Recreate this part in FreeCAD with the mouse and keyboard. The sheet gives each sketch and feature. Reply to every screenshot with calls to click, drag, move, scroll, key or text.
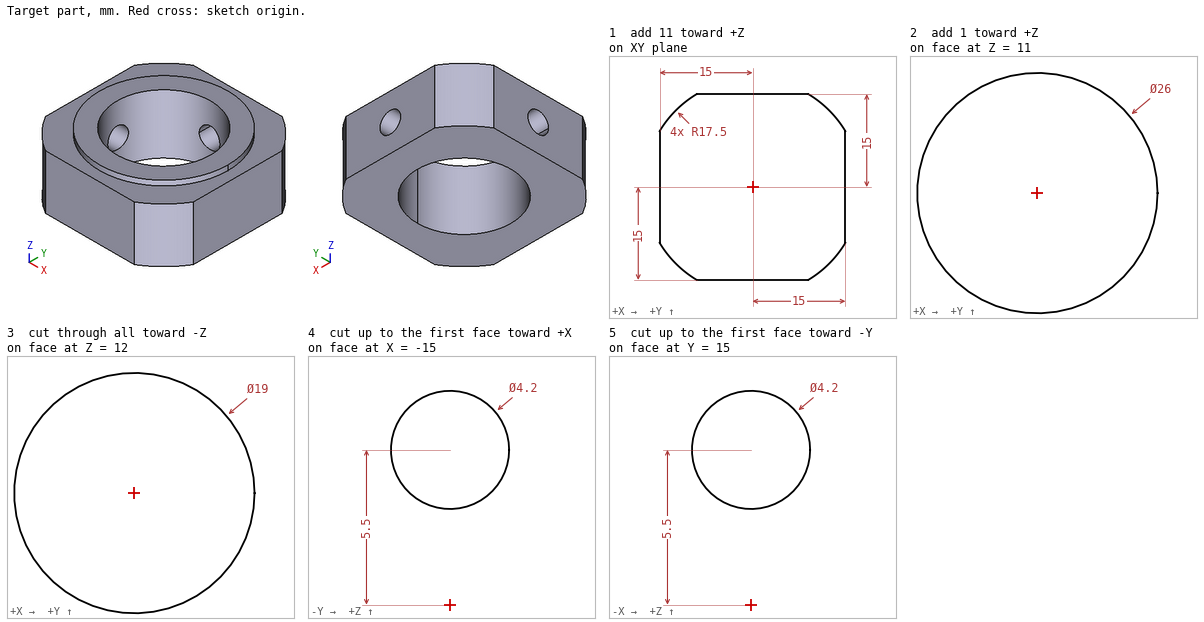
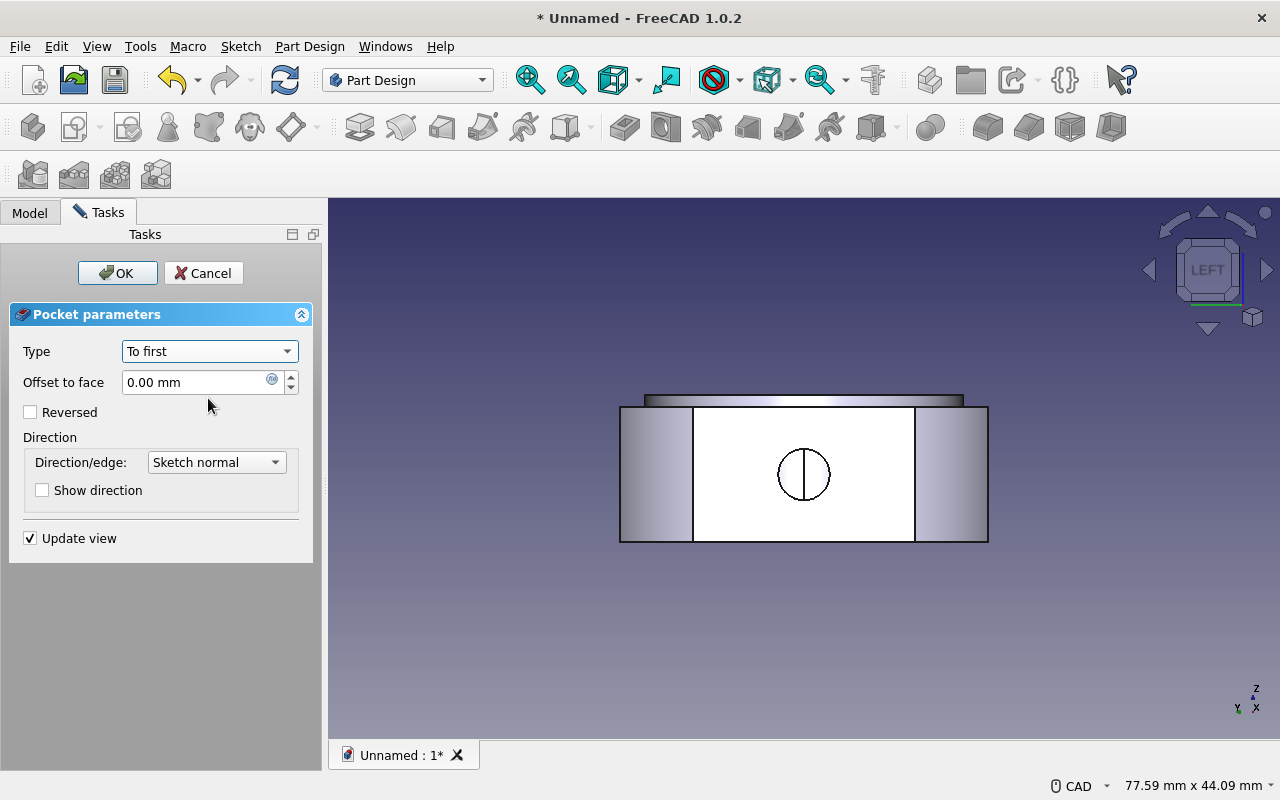
click(118, 273)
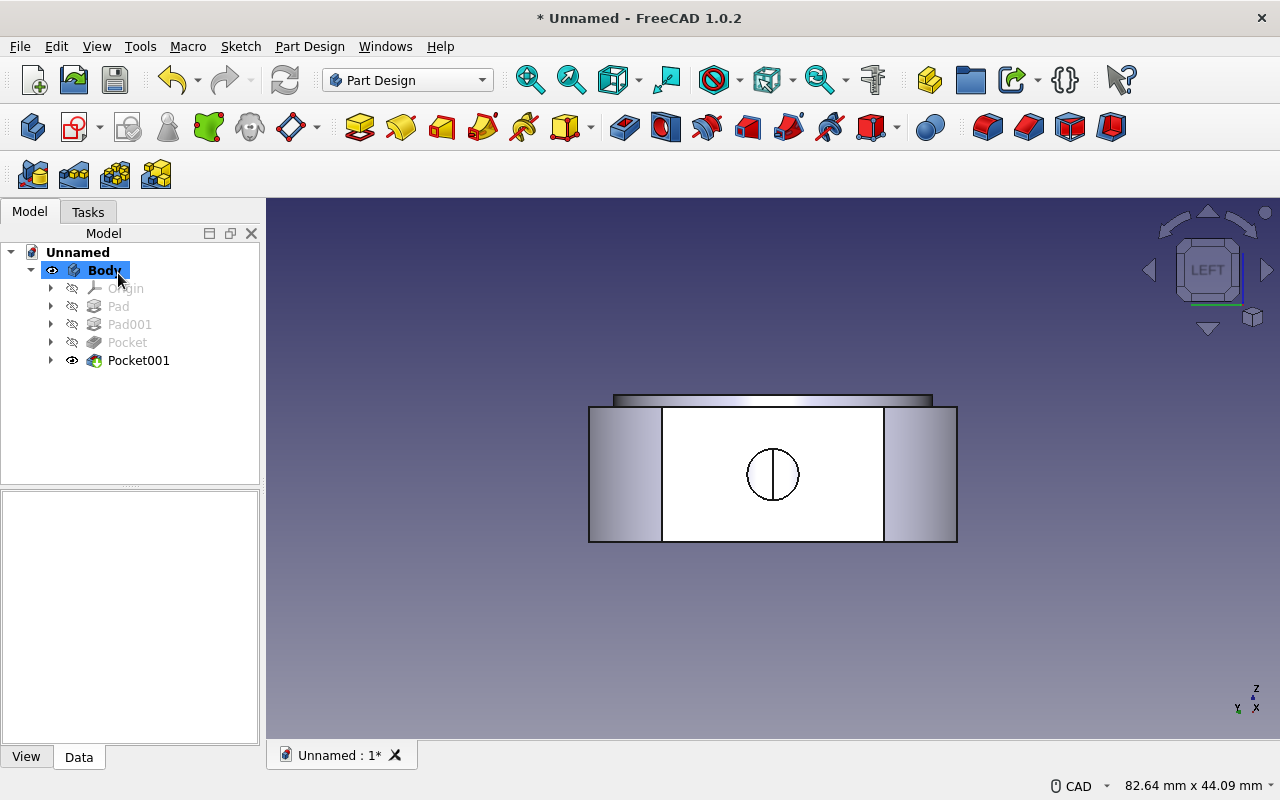
click(531, 80)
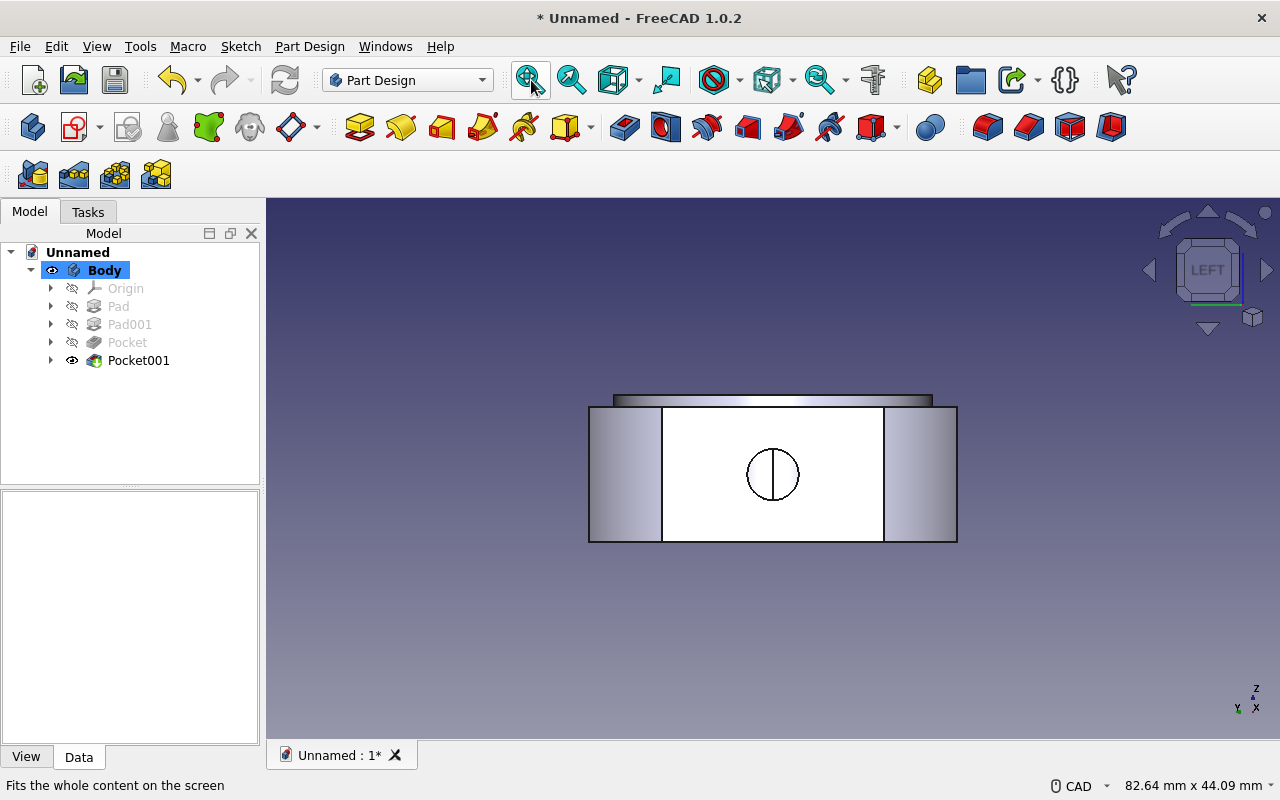
key(4)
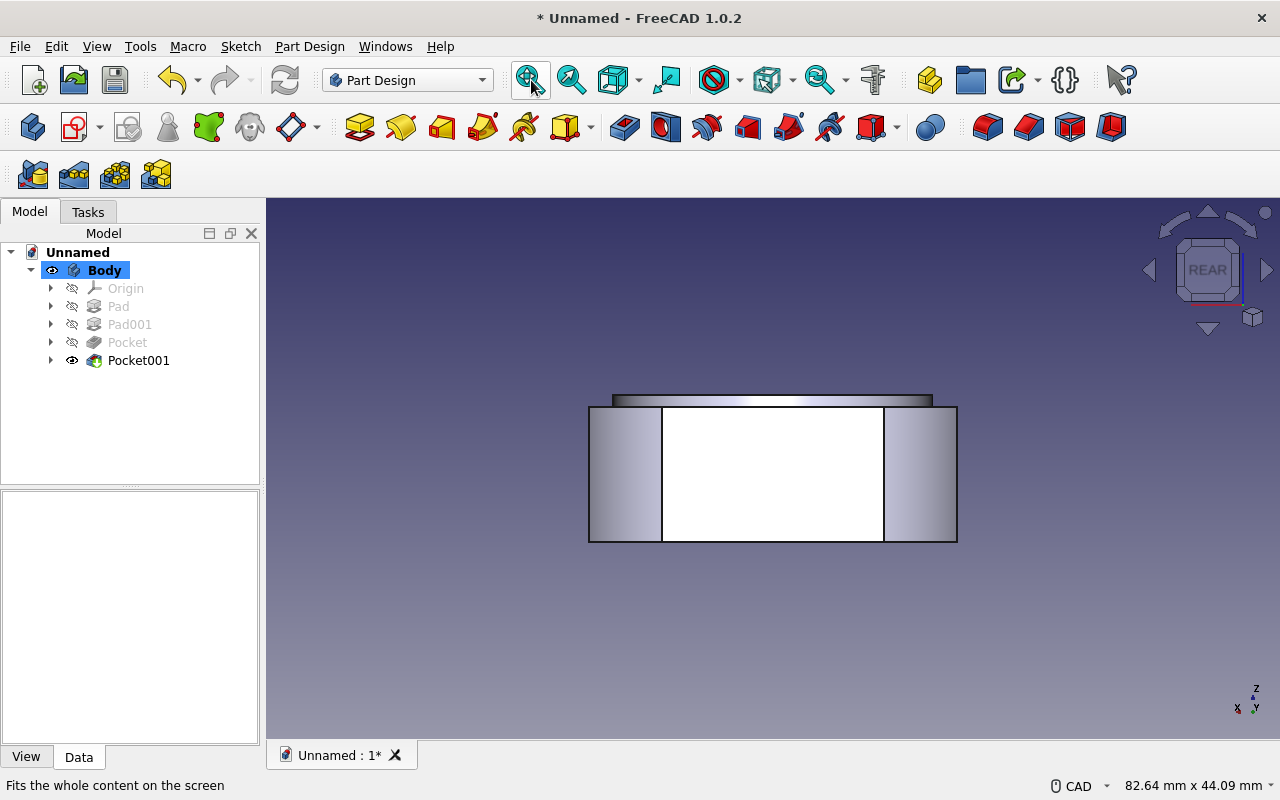
click(531, 80)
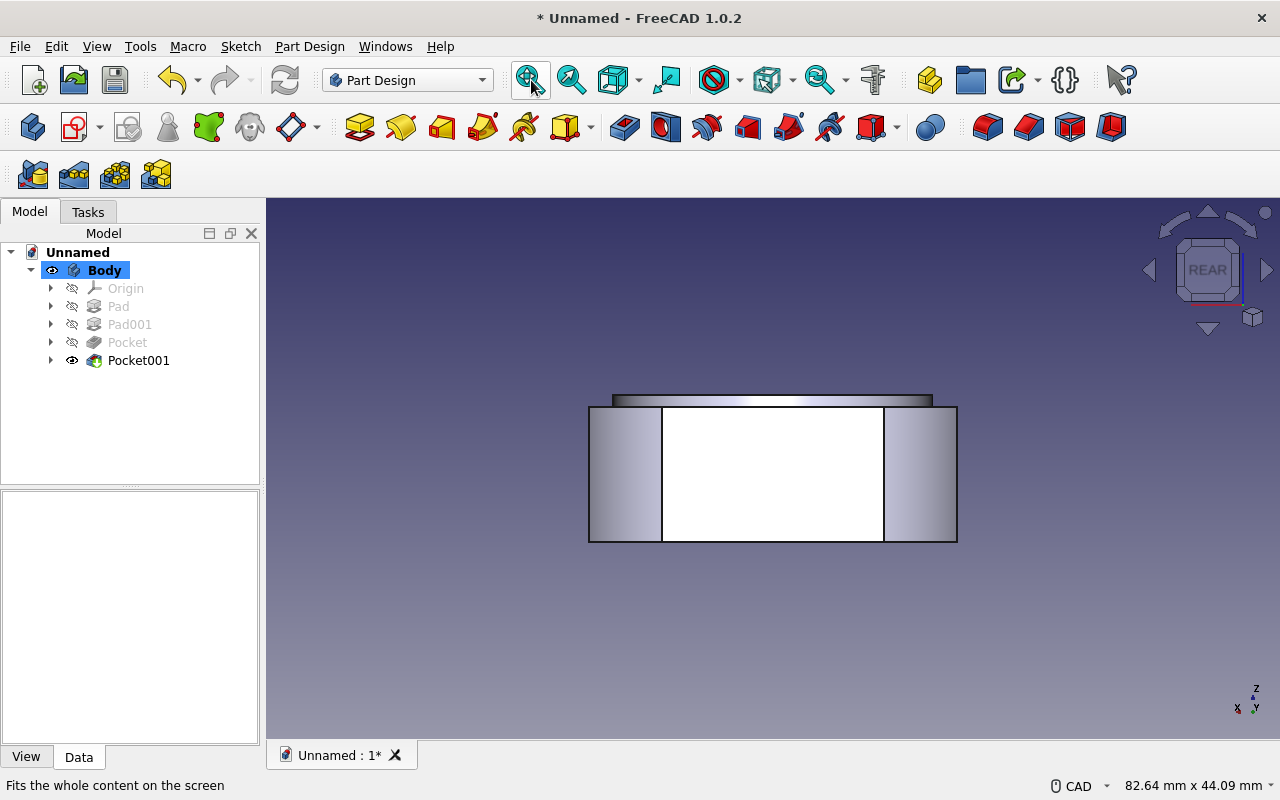
click(741, 474)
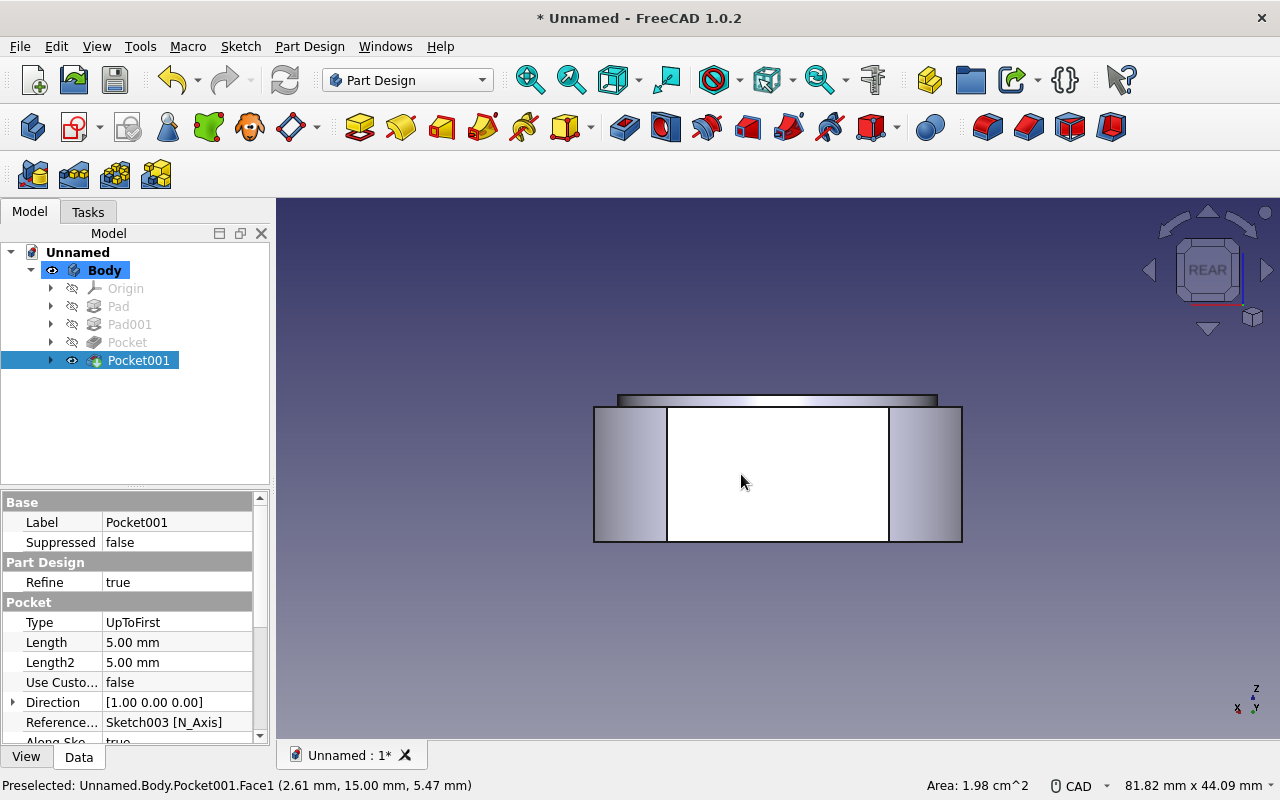
click(74, 128)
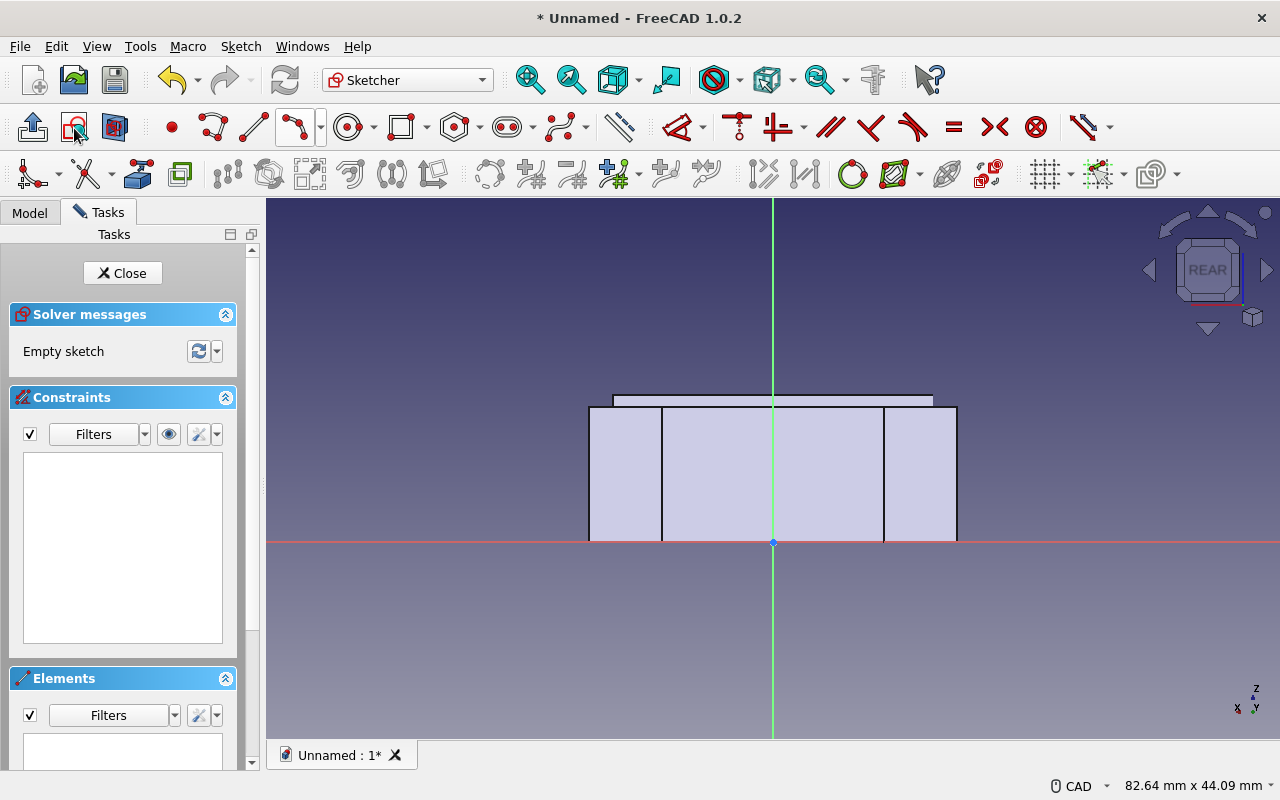
scroll(795, 504, up, 7)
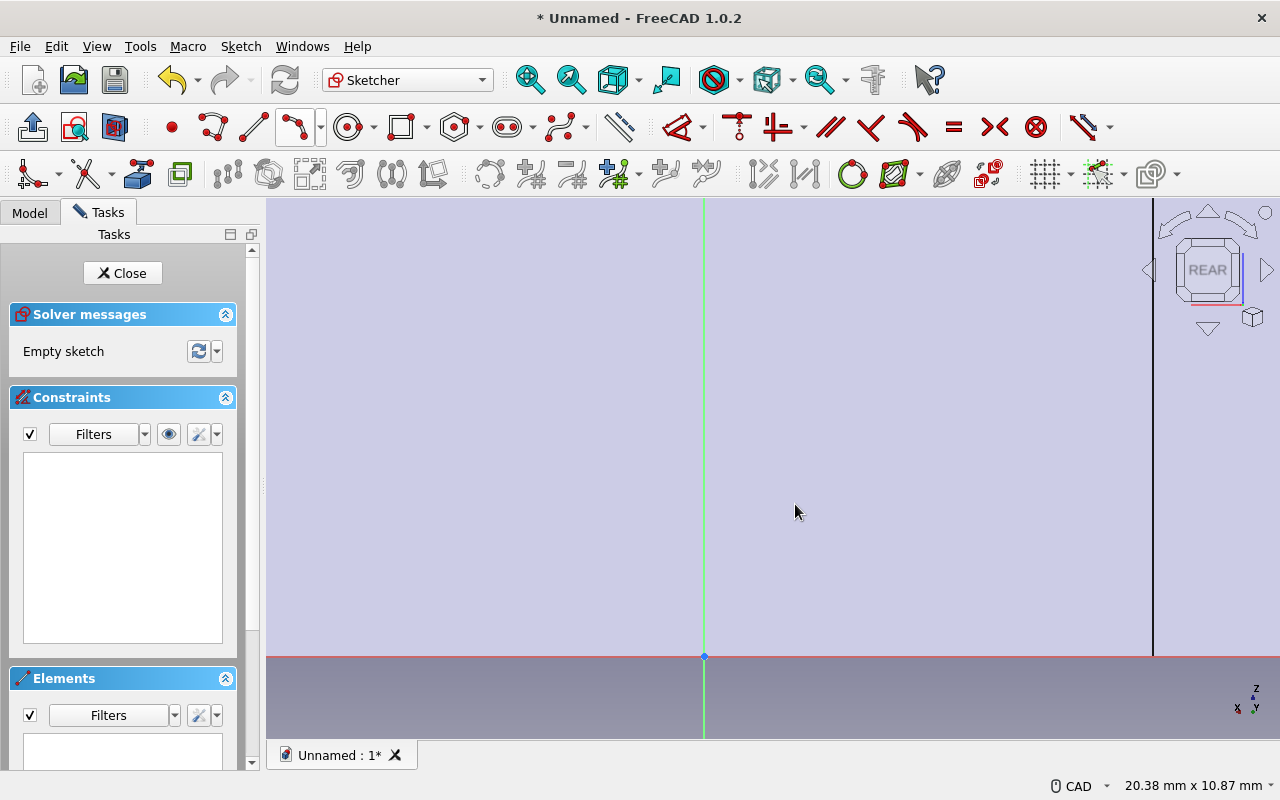
click(348, 128)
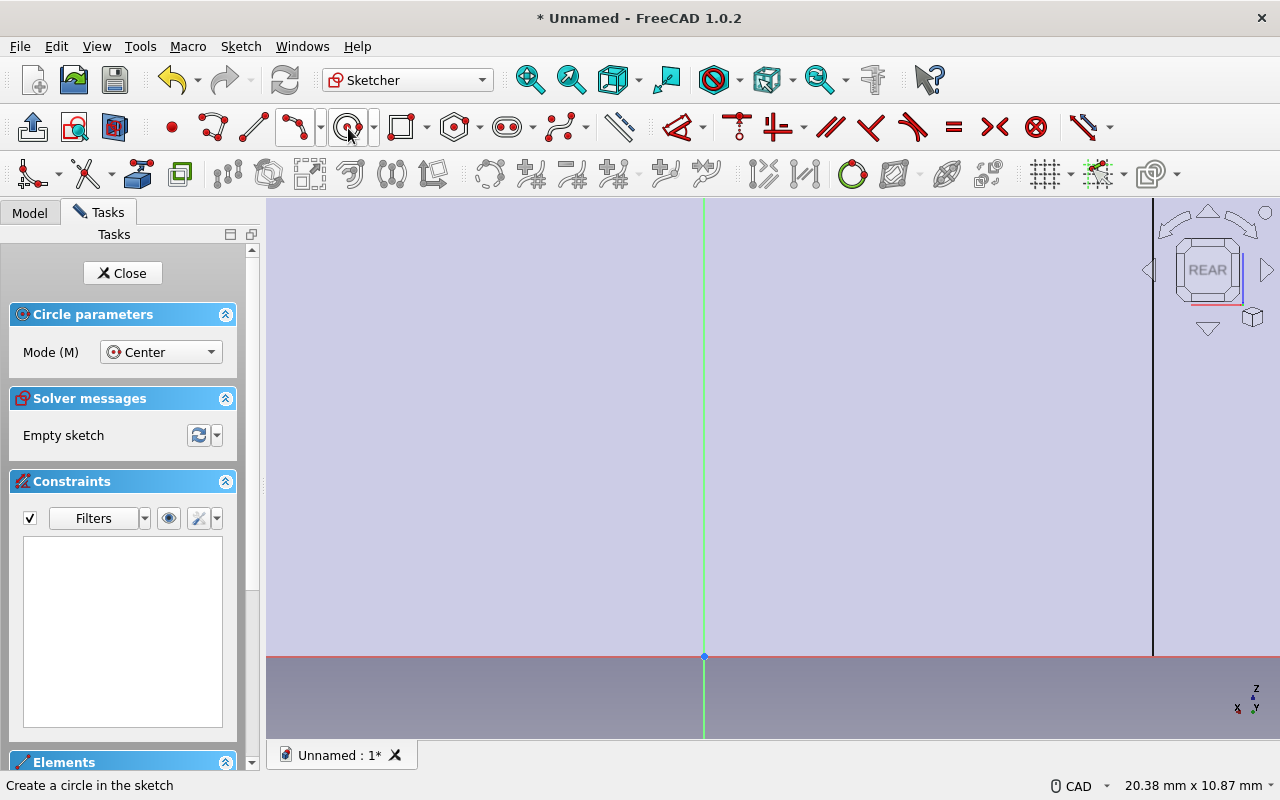
click(704, 383)
click(778, 309)
key(Escape)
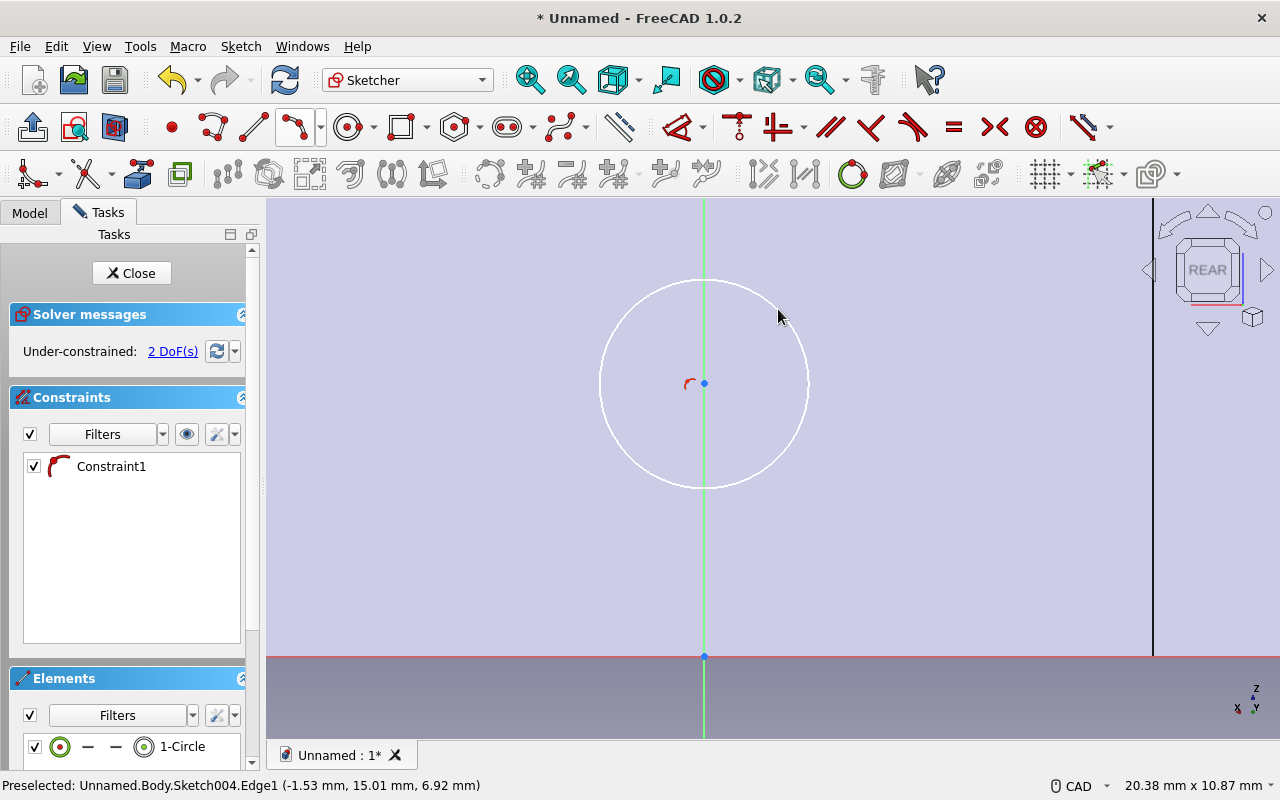
click(676, 128)